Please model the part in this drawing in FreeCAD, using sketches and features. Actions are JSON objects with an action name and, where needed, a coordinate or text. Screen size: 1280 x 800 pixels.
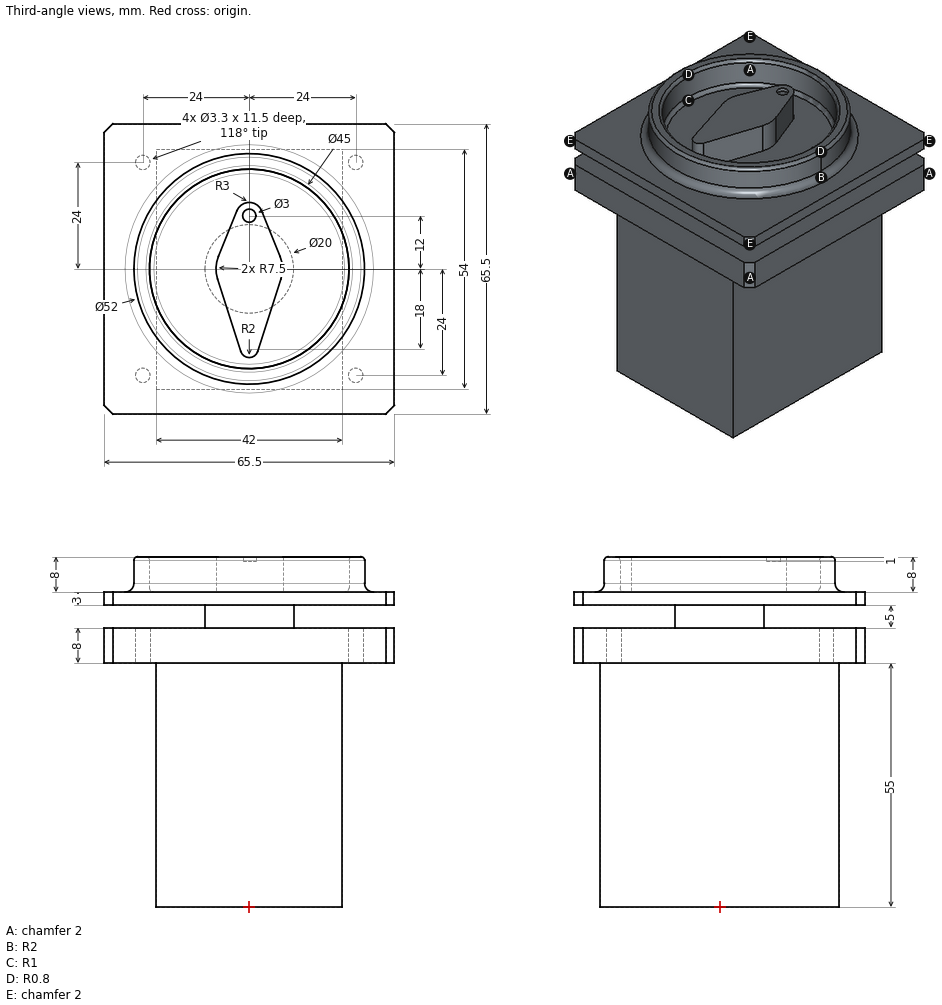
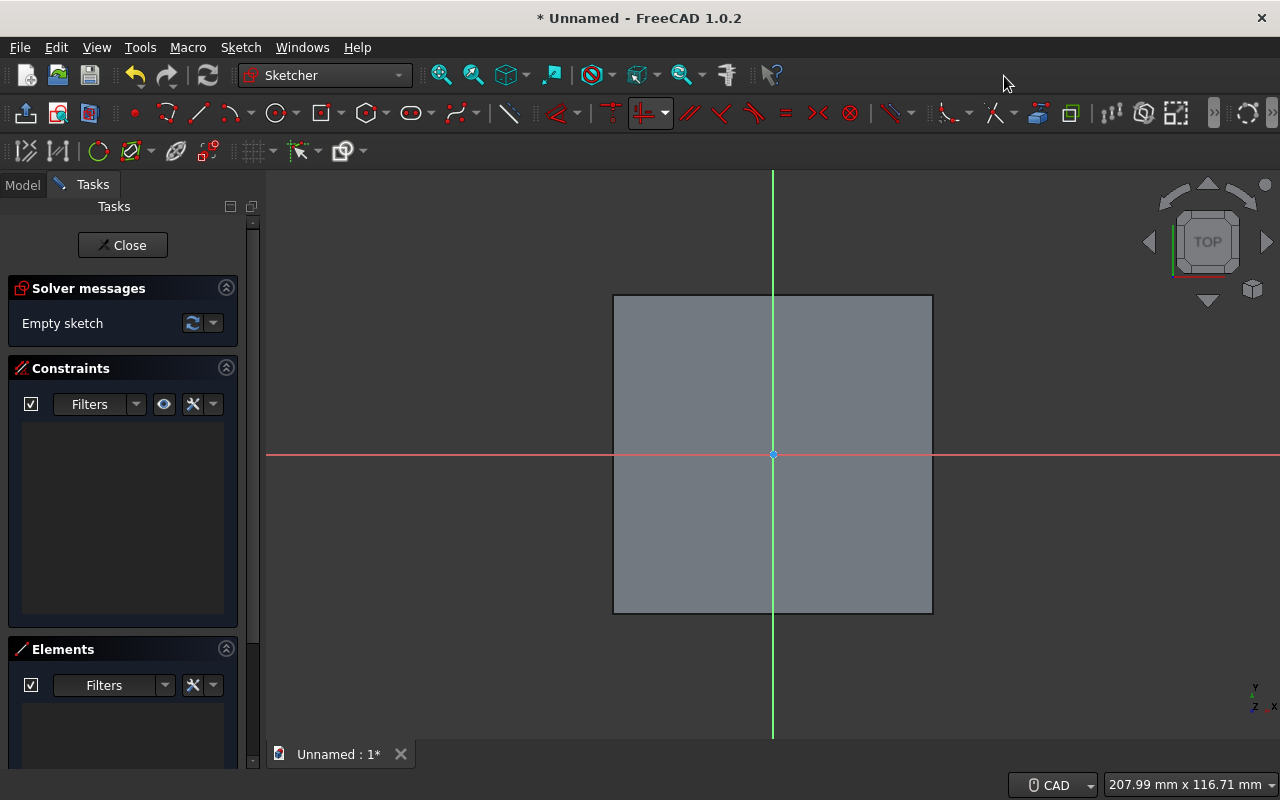
{"action": "scroll", "coordinate": [912, 455], "scroll_direction": "up", "scroll_amount": 2}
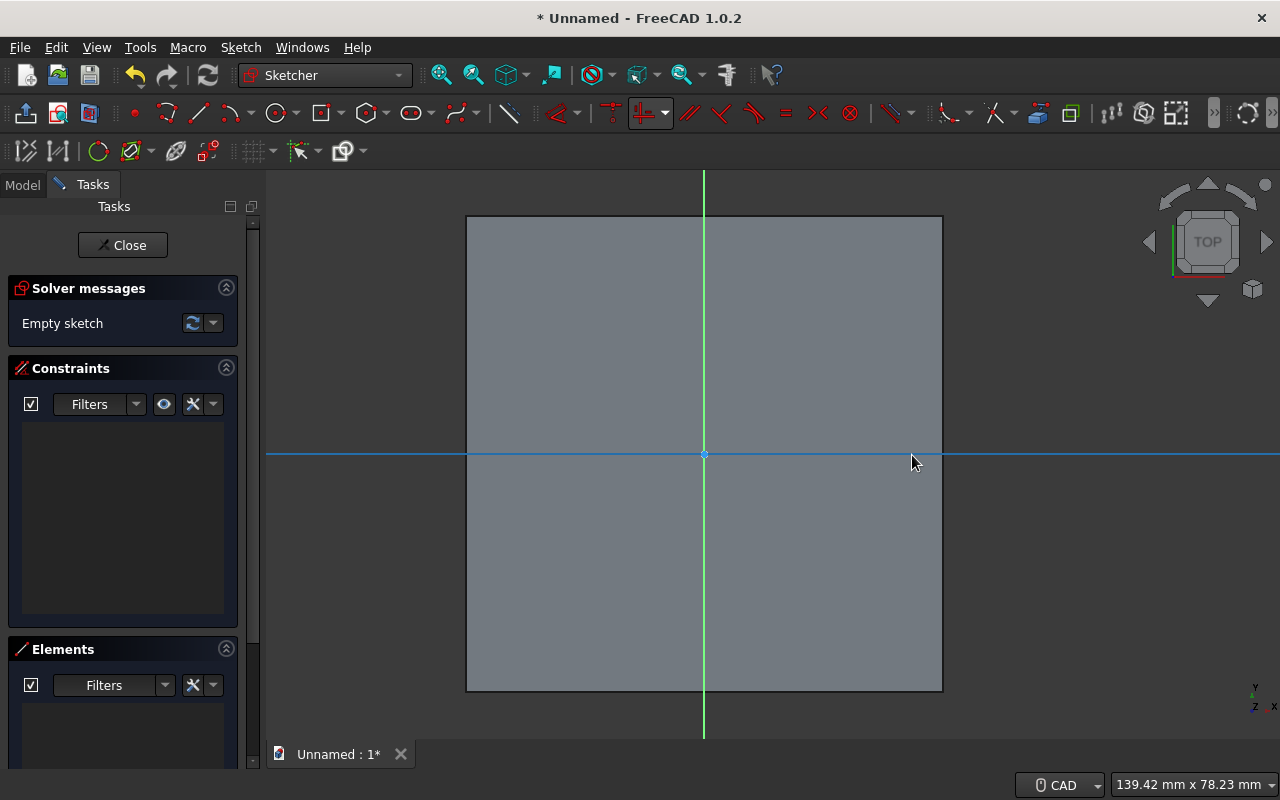
{"action": "left_click", "coordinate": [276, 114]}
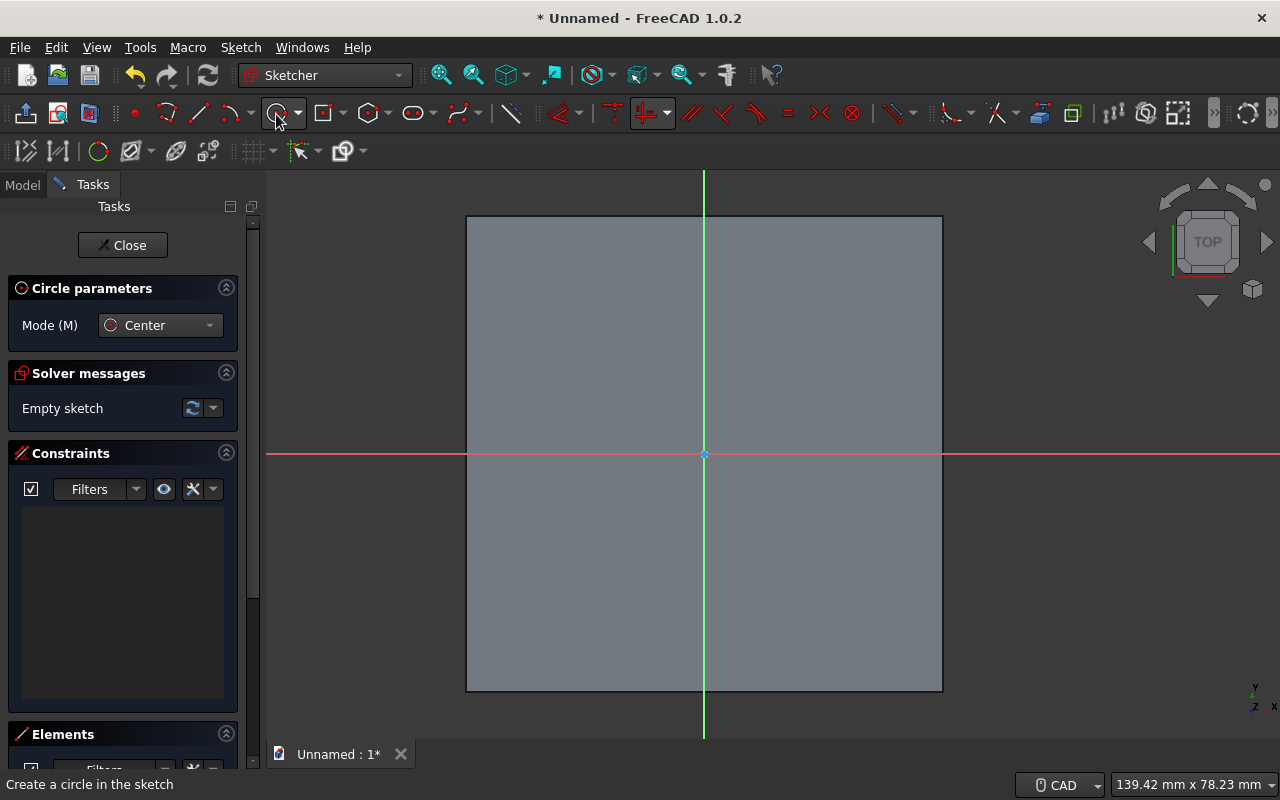
{"action": "left_click", "coordinate": [704, 454]}
{"action": "mouse_move", "coordinate": [838, 320]}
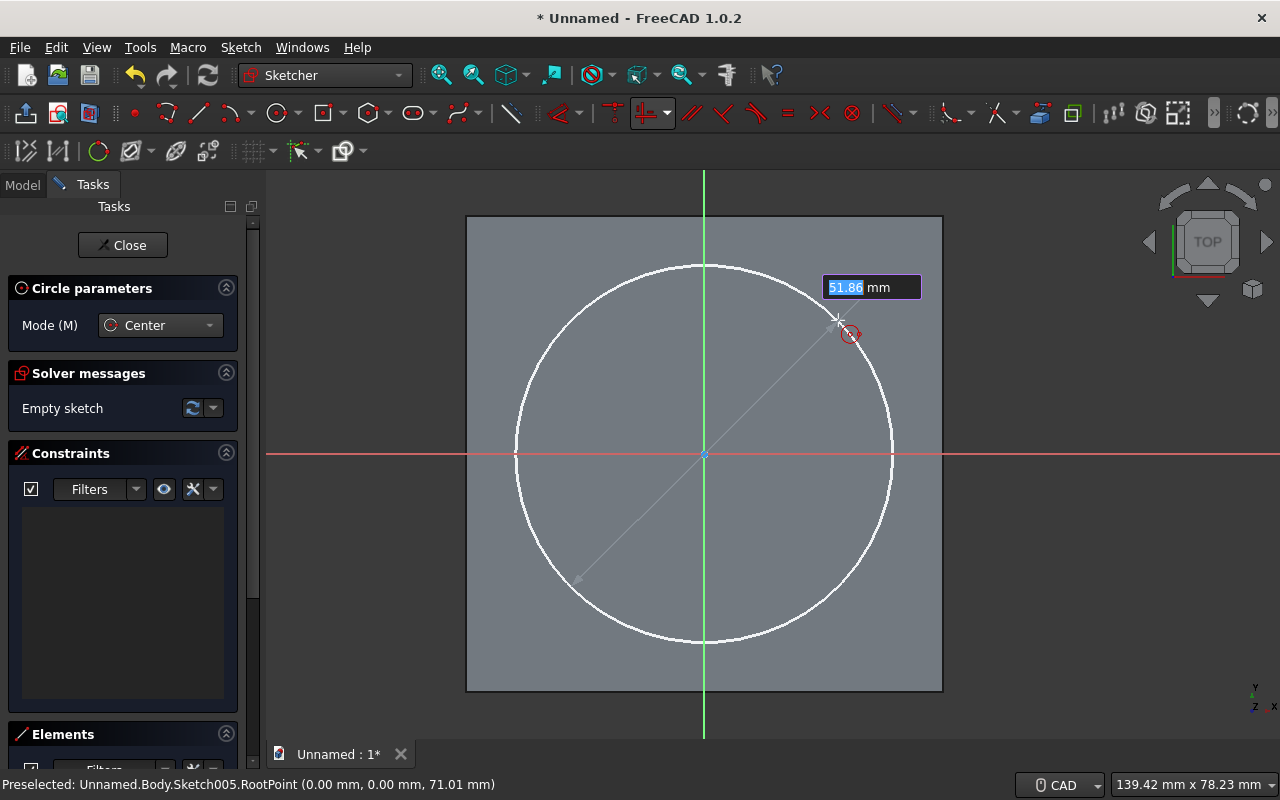
{"action": "type", "text": "52"}
{"action": "key", "text": "Return"}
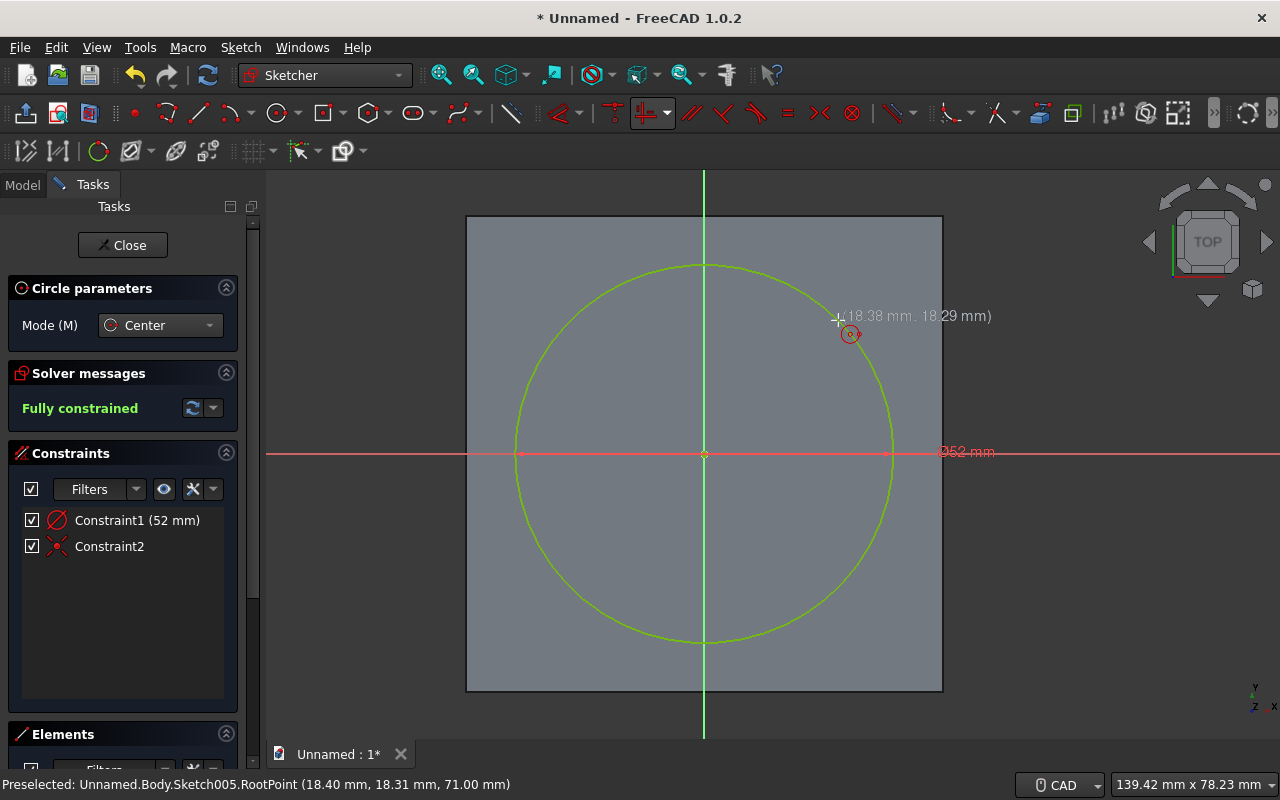
{"action": "left_click", "coordinate": [704, 454]}
{"action": "mouse_move", "coordinate": [820, 338]}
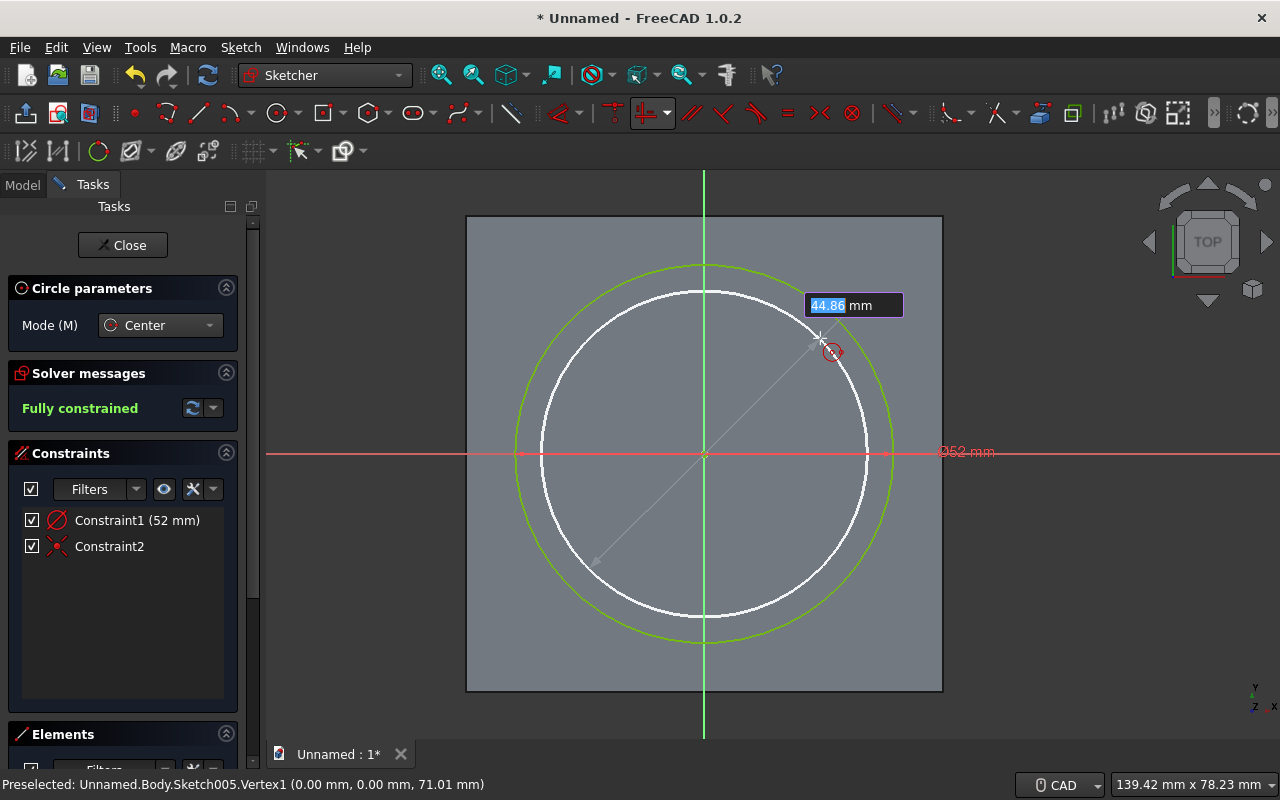
{"action": "type", "text": "45"}
{"action": "key", "text": "Return"}
{"action": "key", "text": "Escape"}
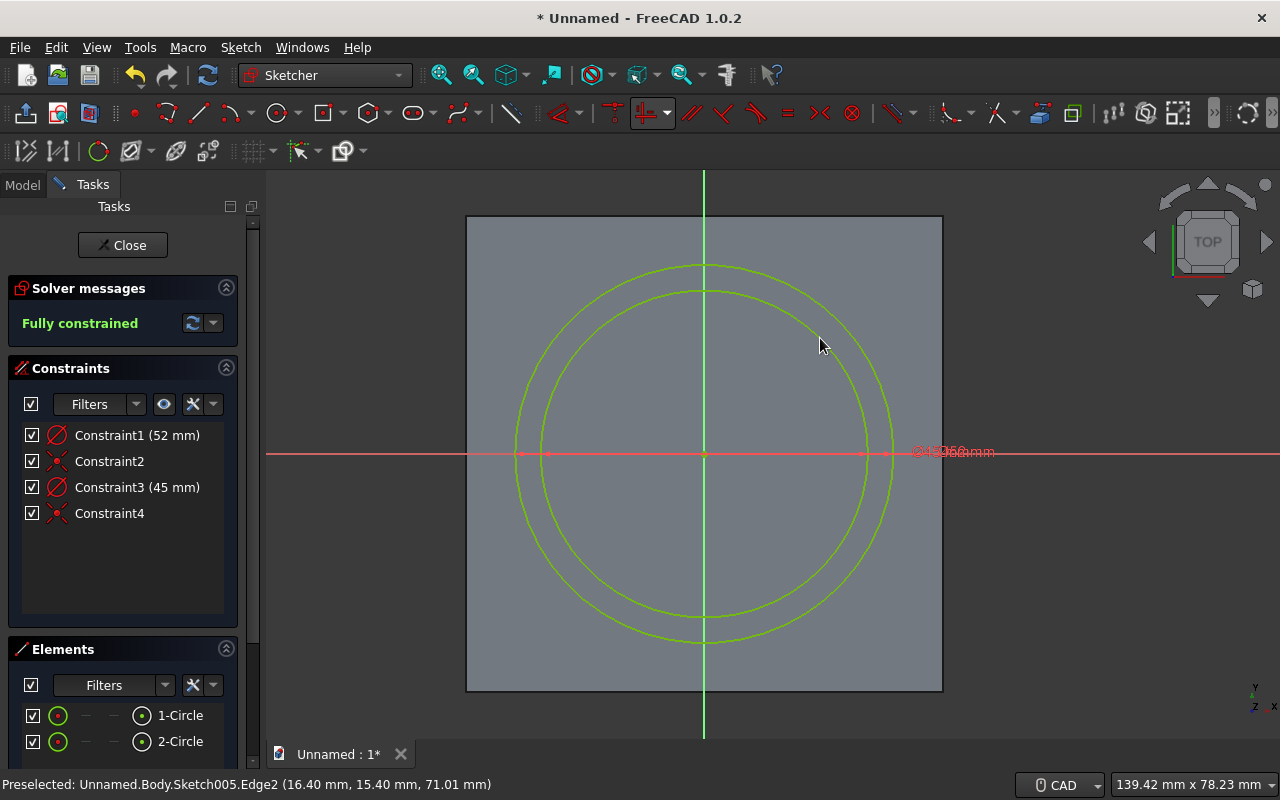
{"action": "left_click", "coordinate": [123, 245]}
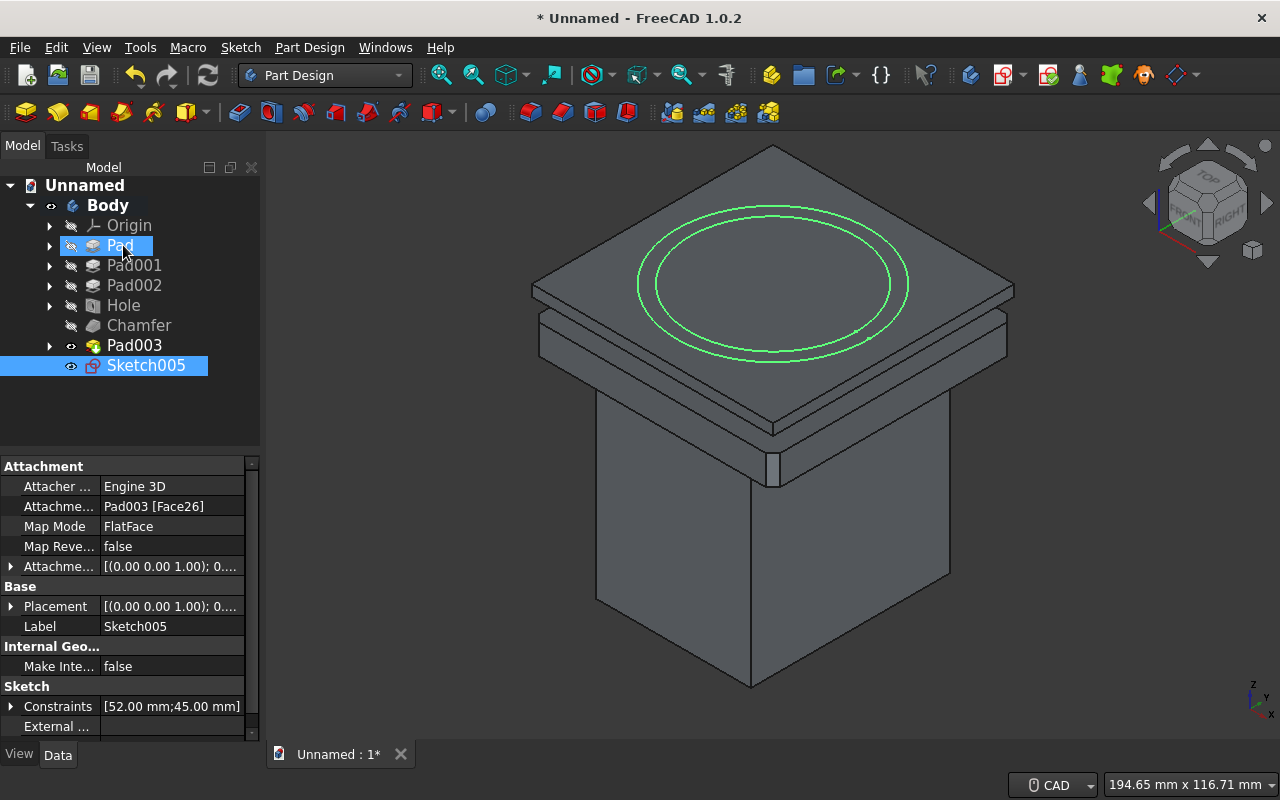
{"action": "left_click", "coordinate": [26, 112]}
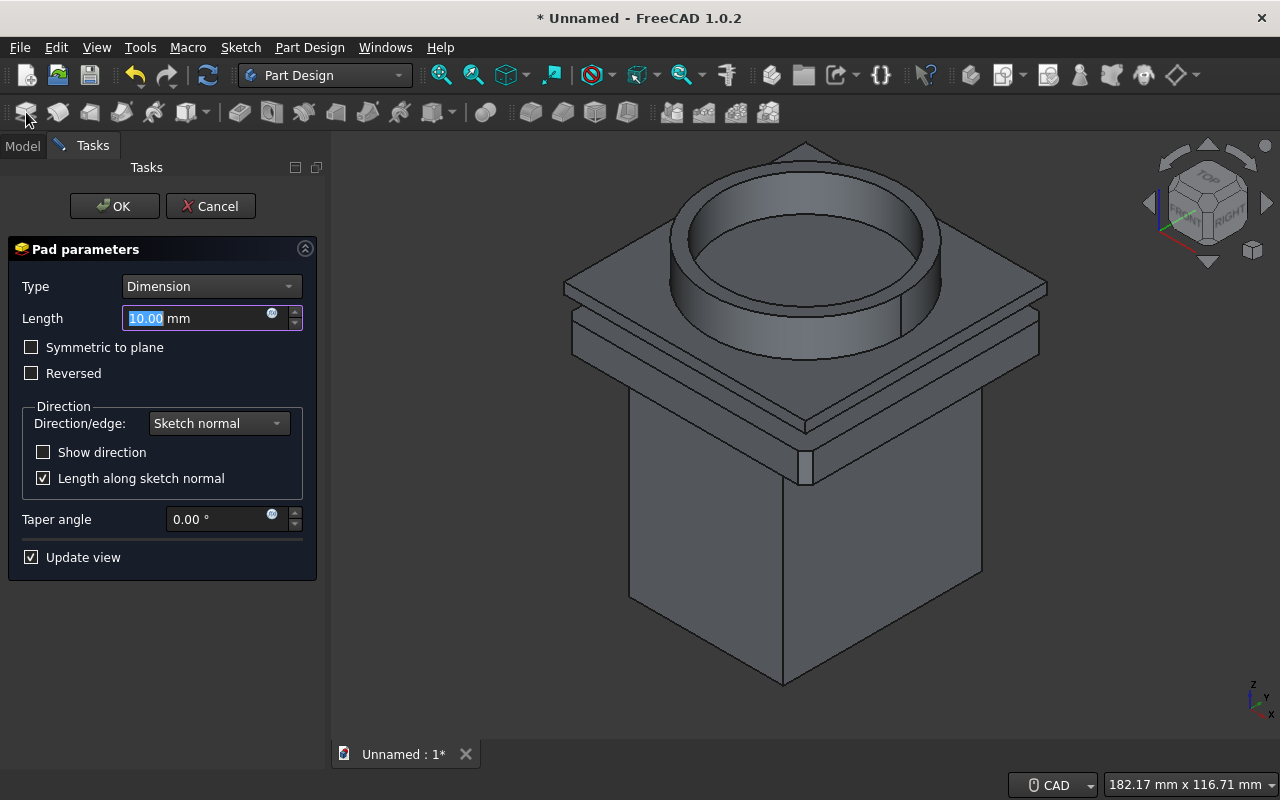
{"action": "type", "text": "8"}
{"action": "key", "text": "Tab"}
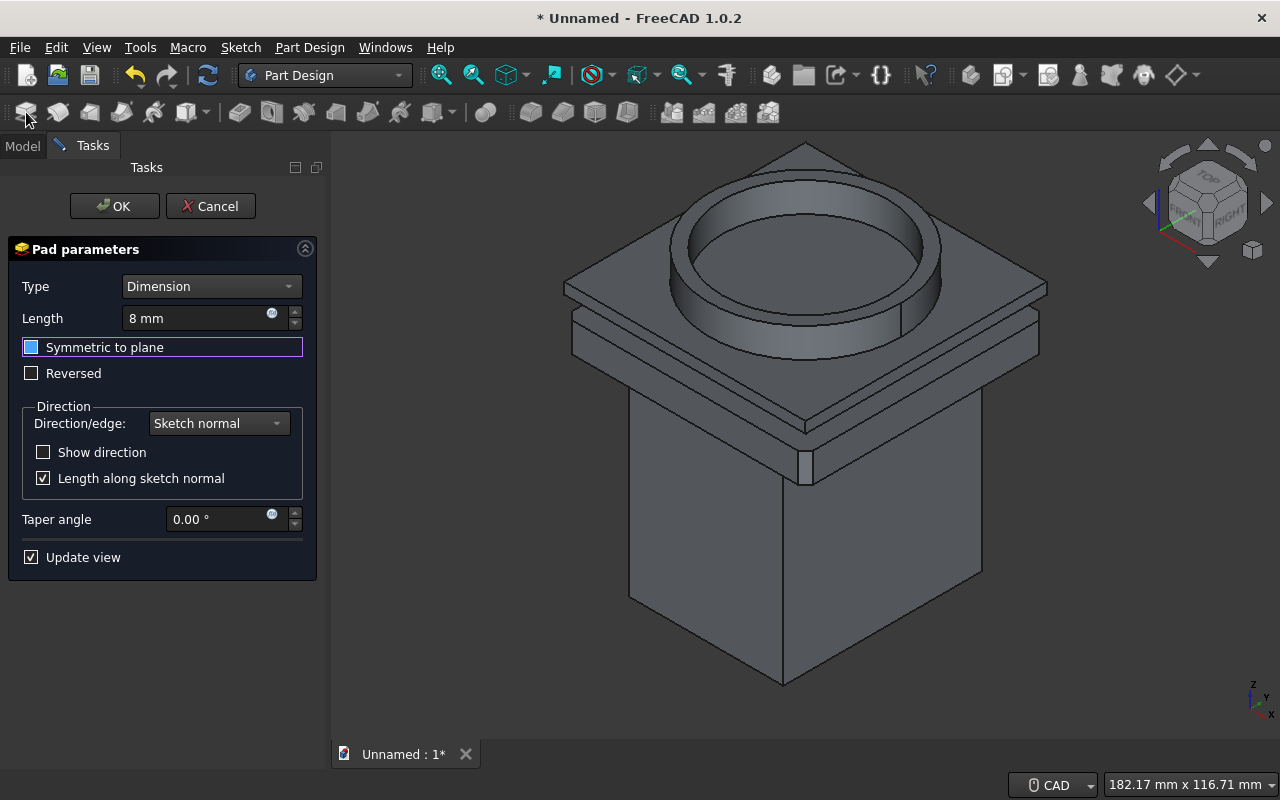
{"action": "left_click", "coordinate": [115, 206]}